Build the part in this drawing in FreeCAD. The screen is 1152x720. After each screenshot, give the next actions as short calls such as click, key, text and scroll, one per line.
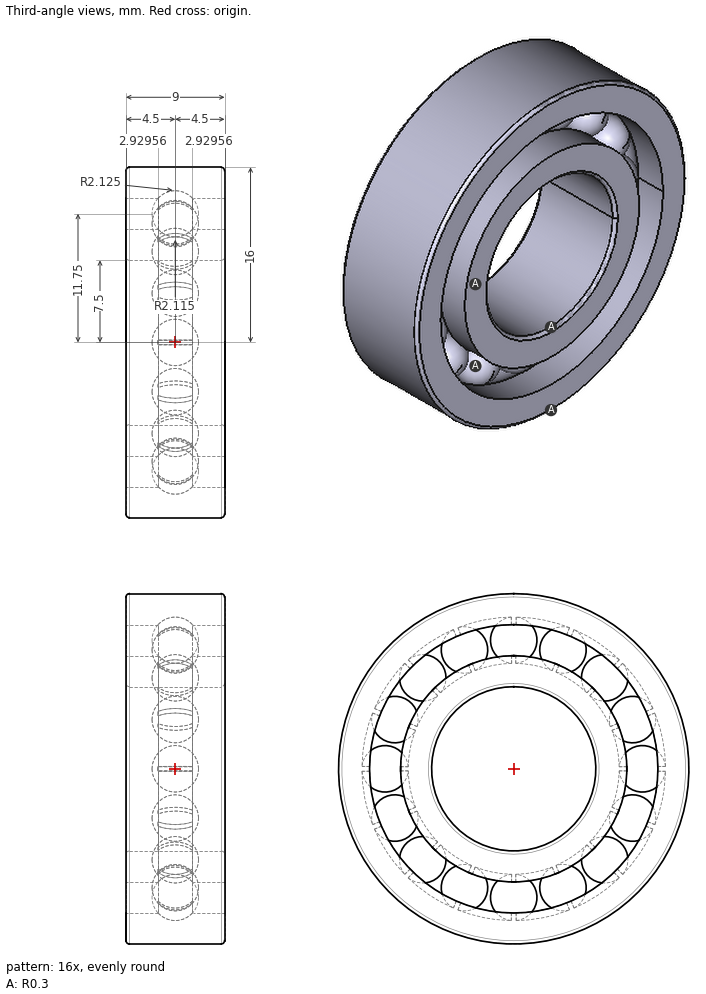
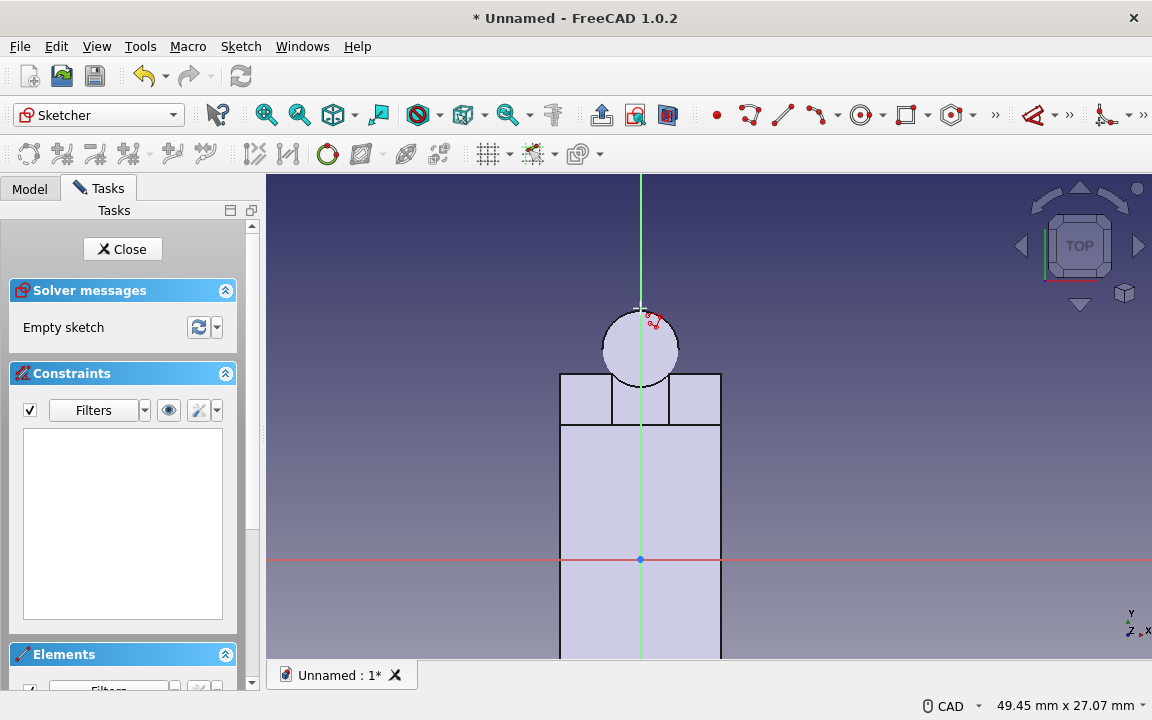
click(669, 324)
click(721, 324)
click(721, 273)
click(560, 273)
click(560, 324)
click(612, 324)
right_click(612, 324)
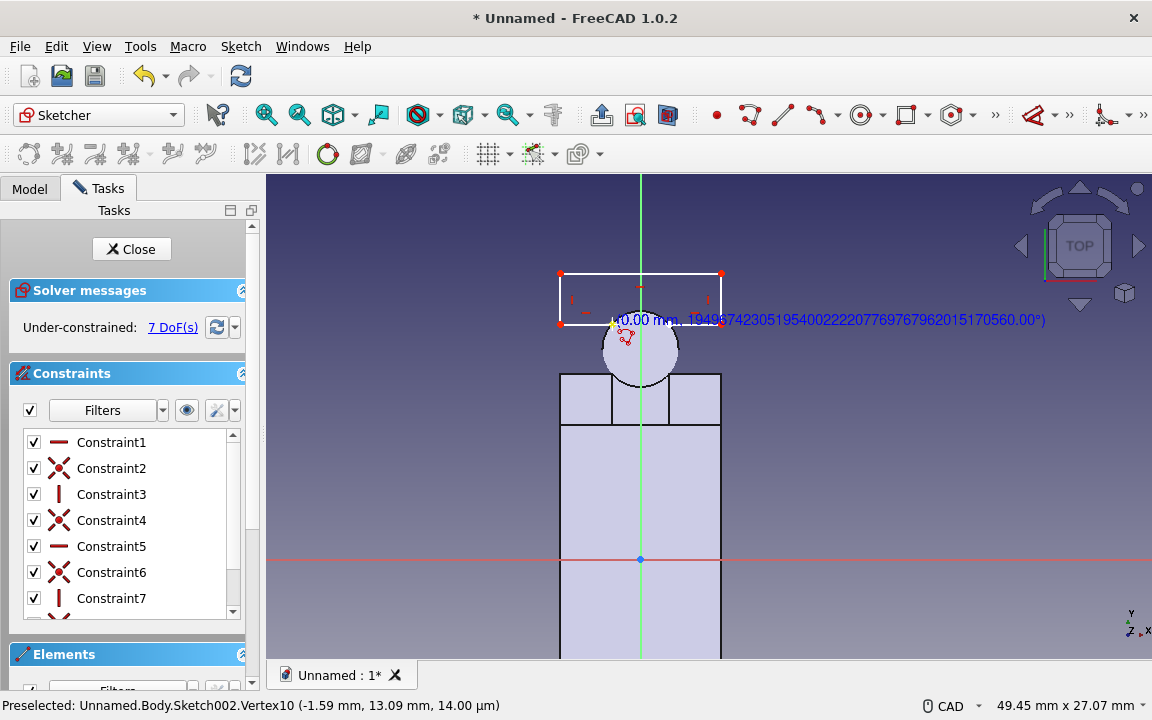
click(816, 116)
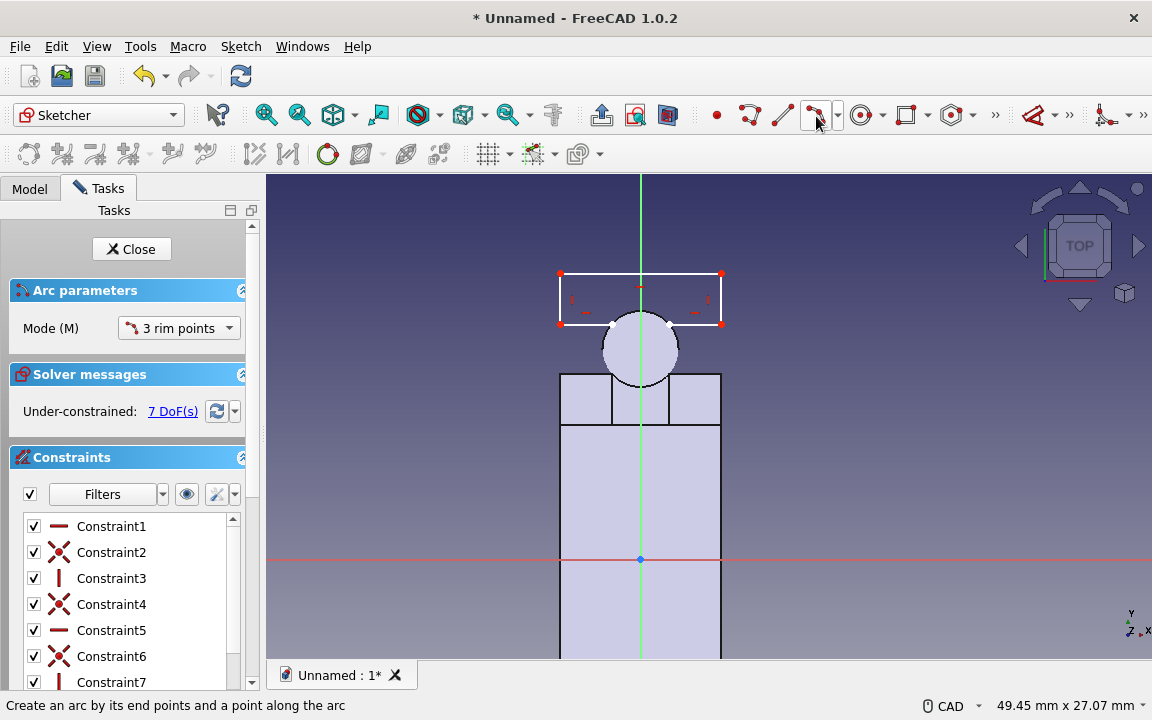
click(612, 325)
click(669, 325)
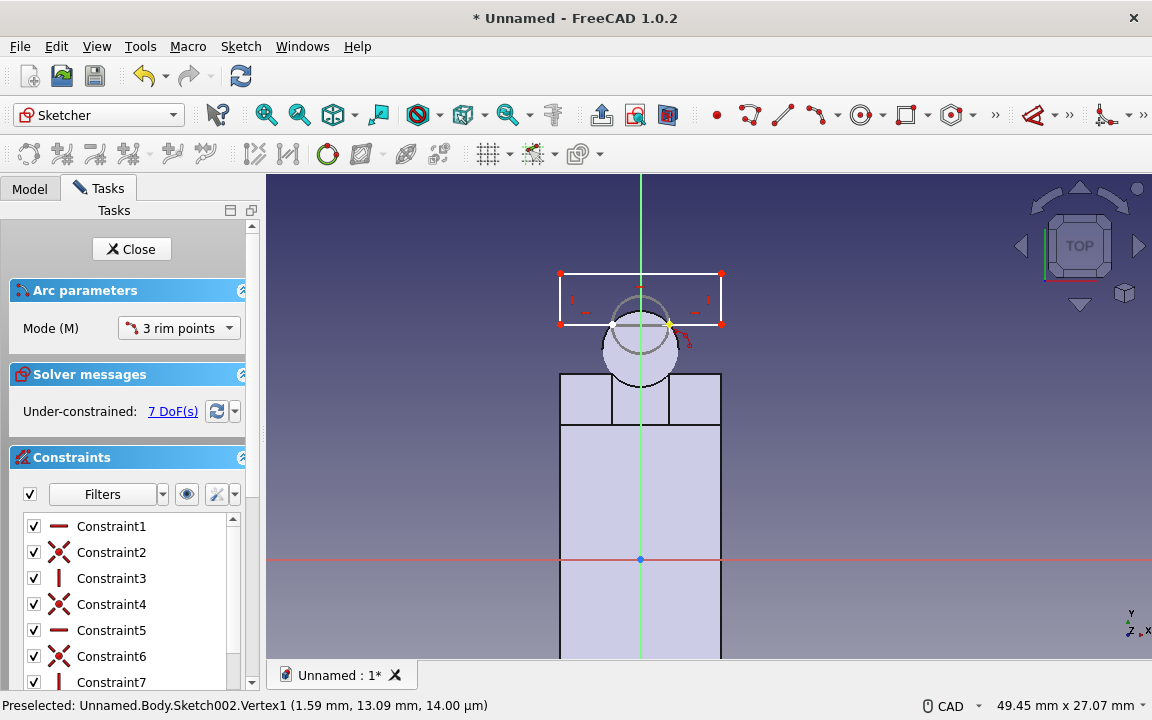
scroll(653, 313, up, 3)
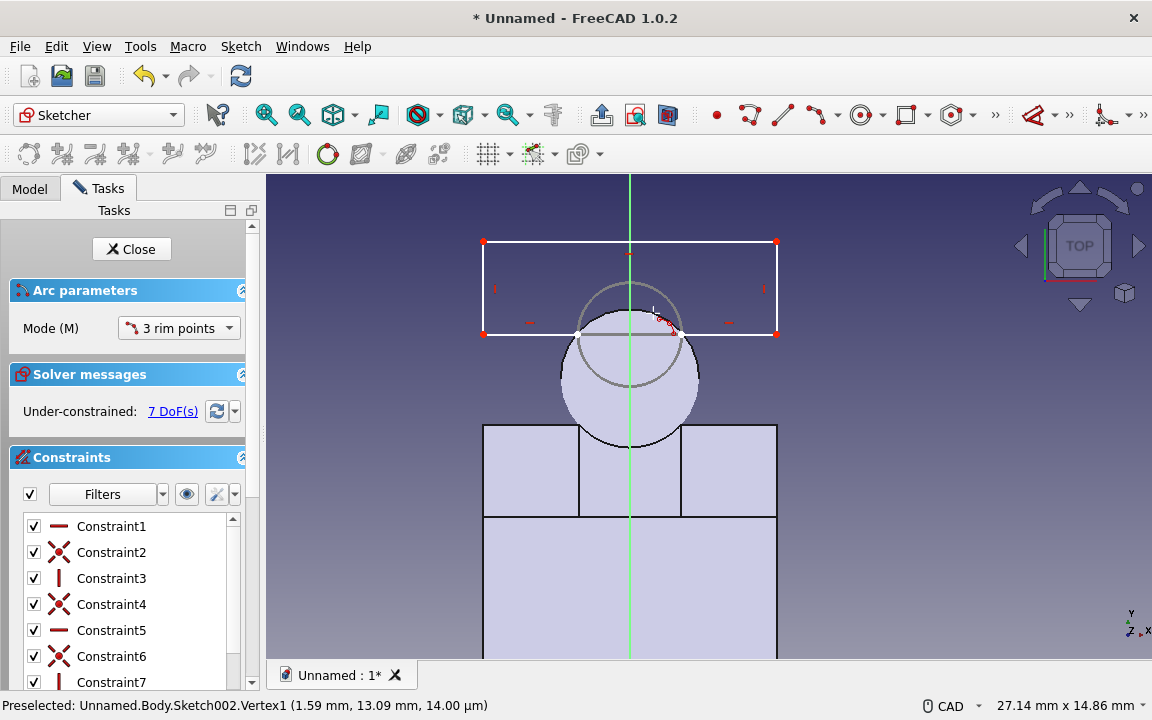
click(653, 313)
key(Escape)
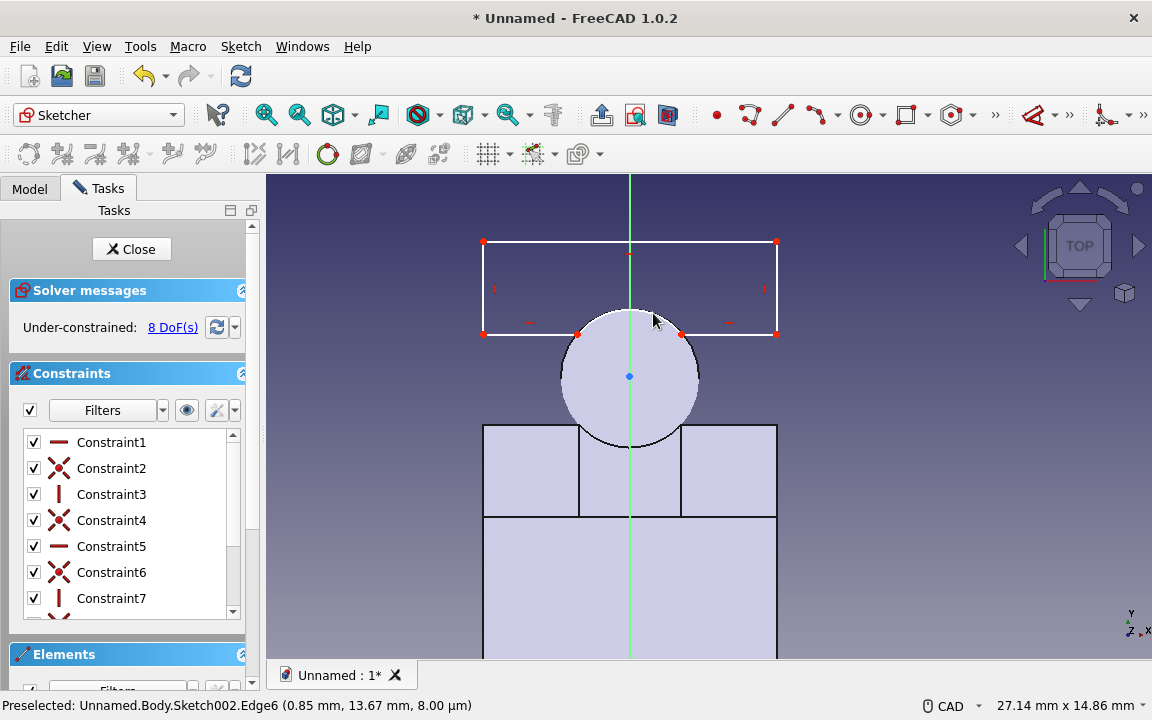
click(630, 377)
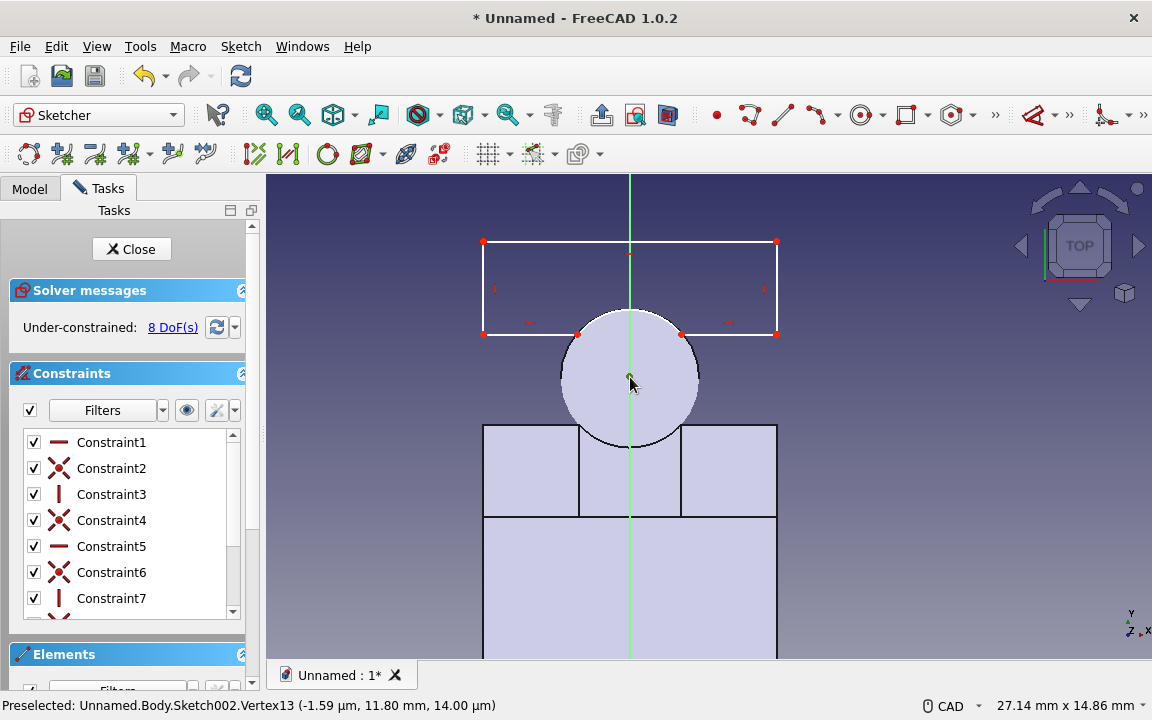
click(630, 600)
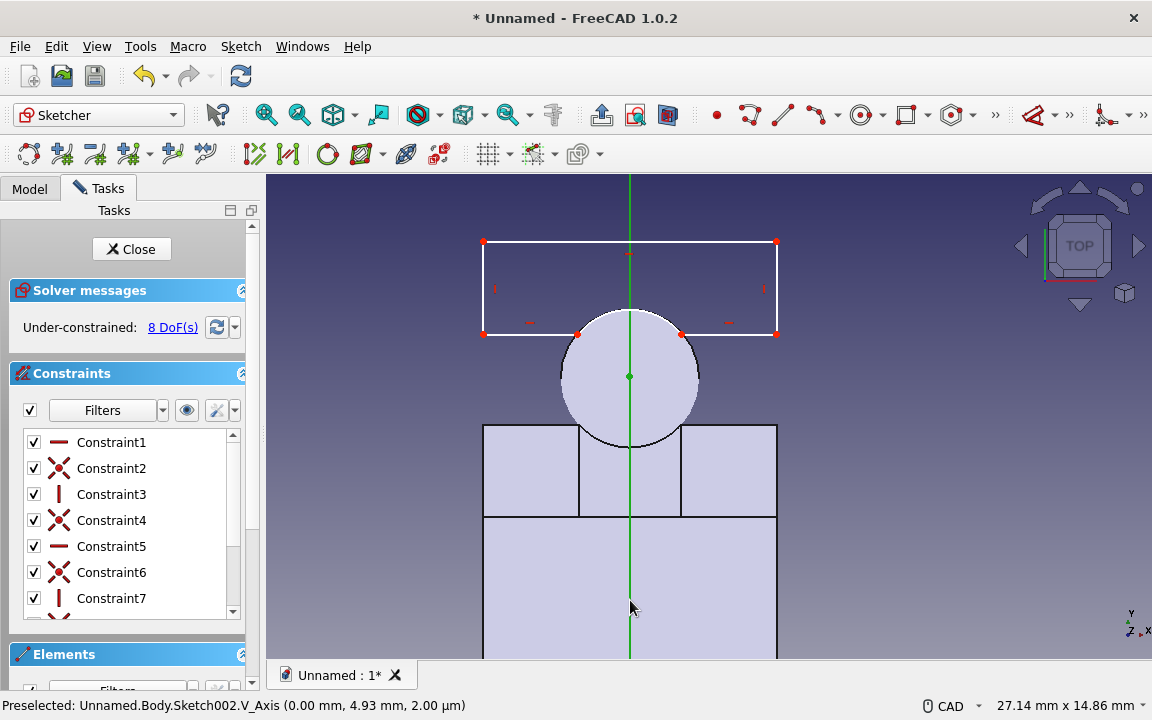
key(c)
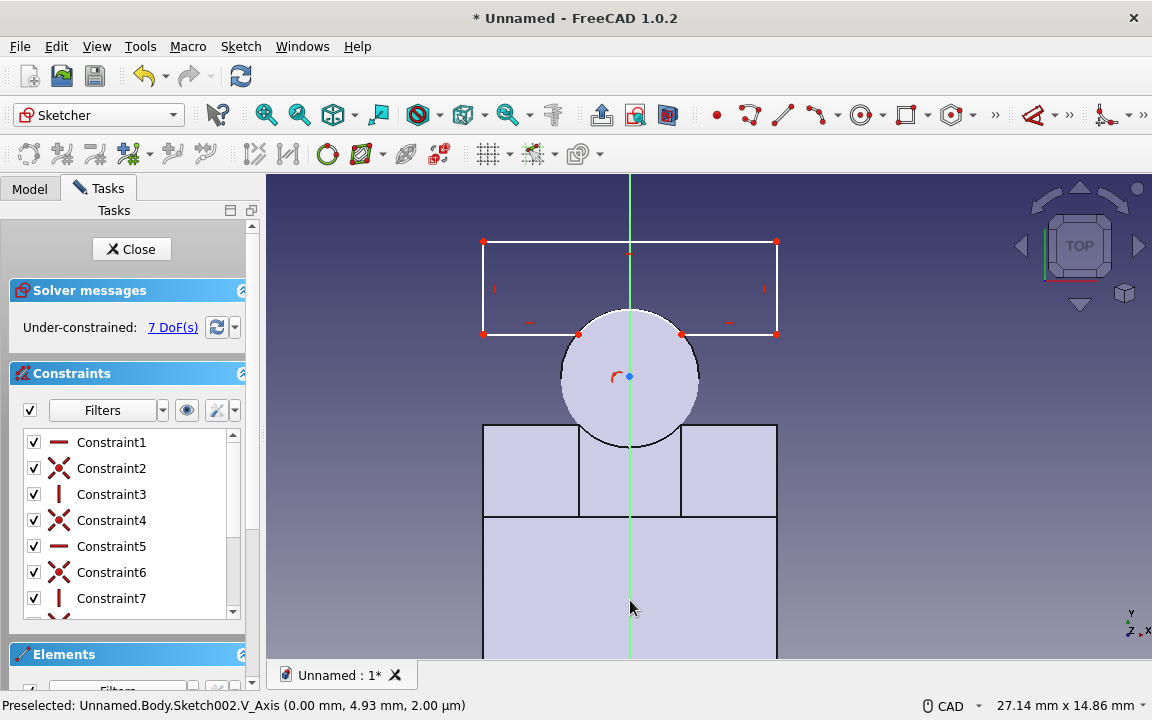
click(1032, 116)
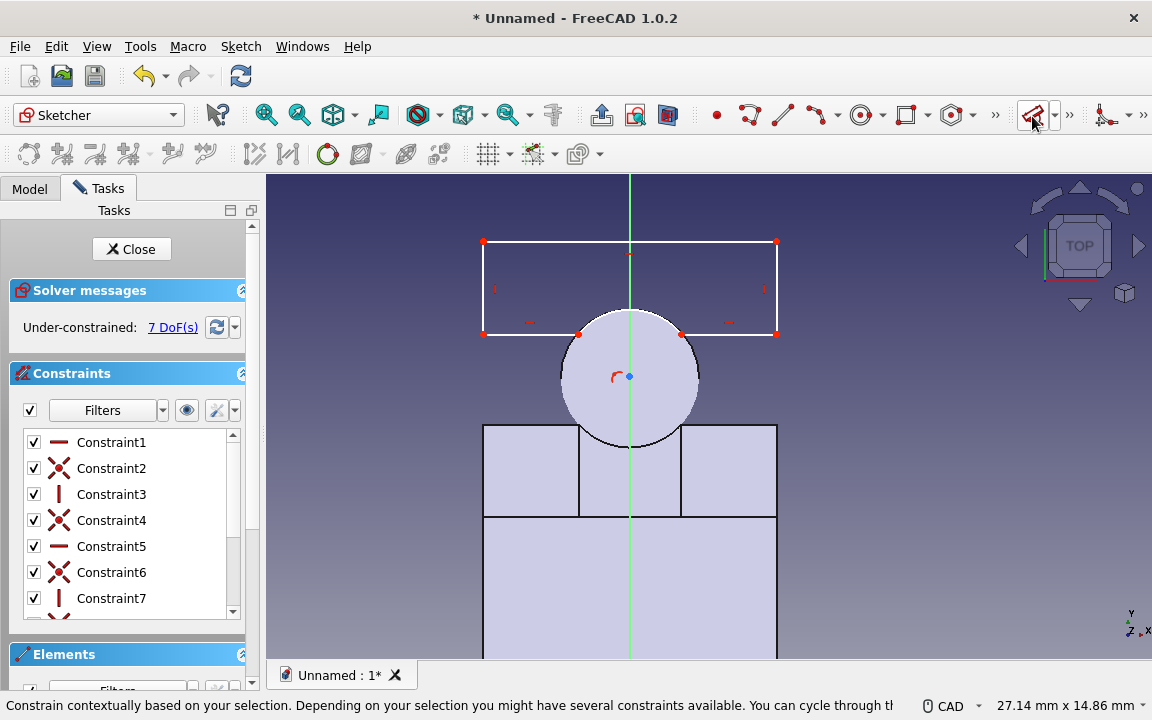
click(653, 314)
click(664, 284)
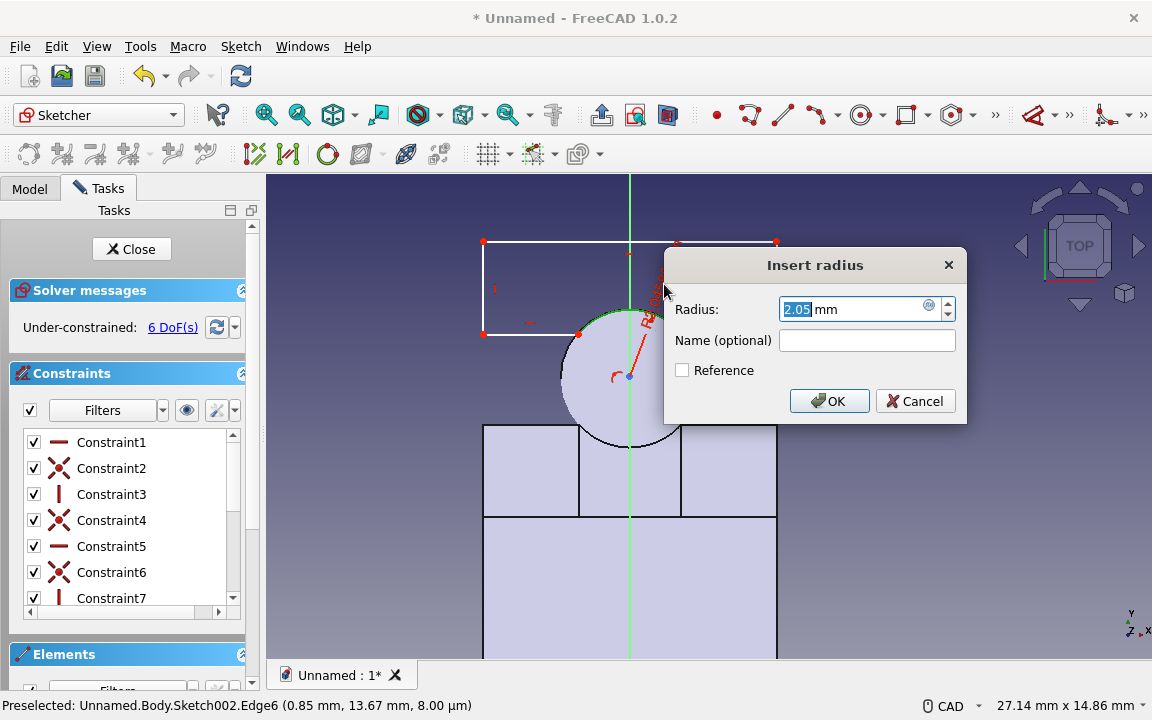
text(2.115)
key(Return)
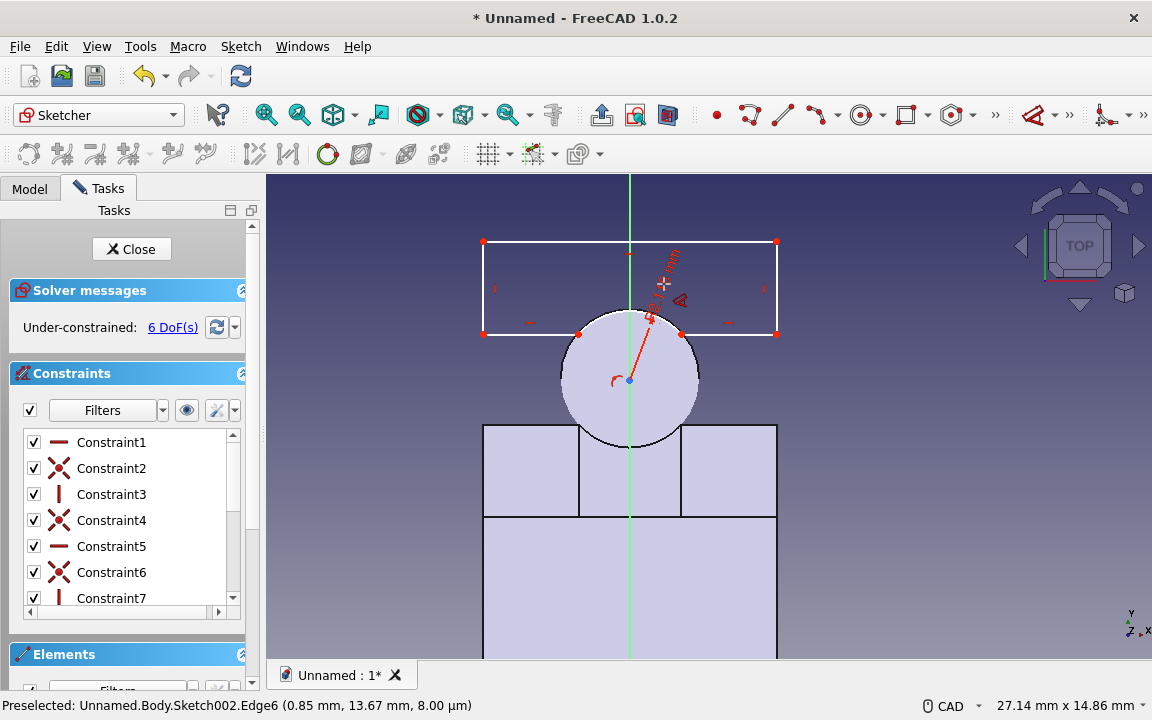
click(689, 242)
click(562, 208)